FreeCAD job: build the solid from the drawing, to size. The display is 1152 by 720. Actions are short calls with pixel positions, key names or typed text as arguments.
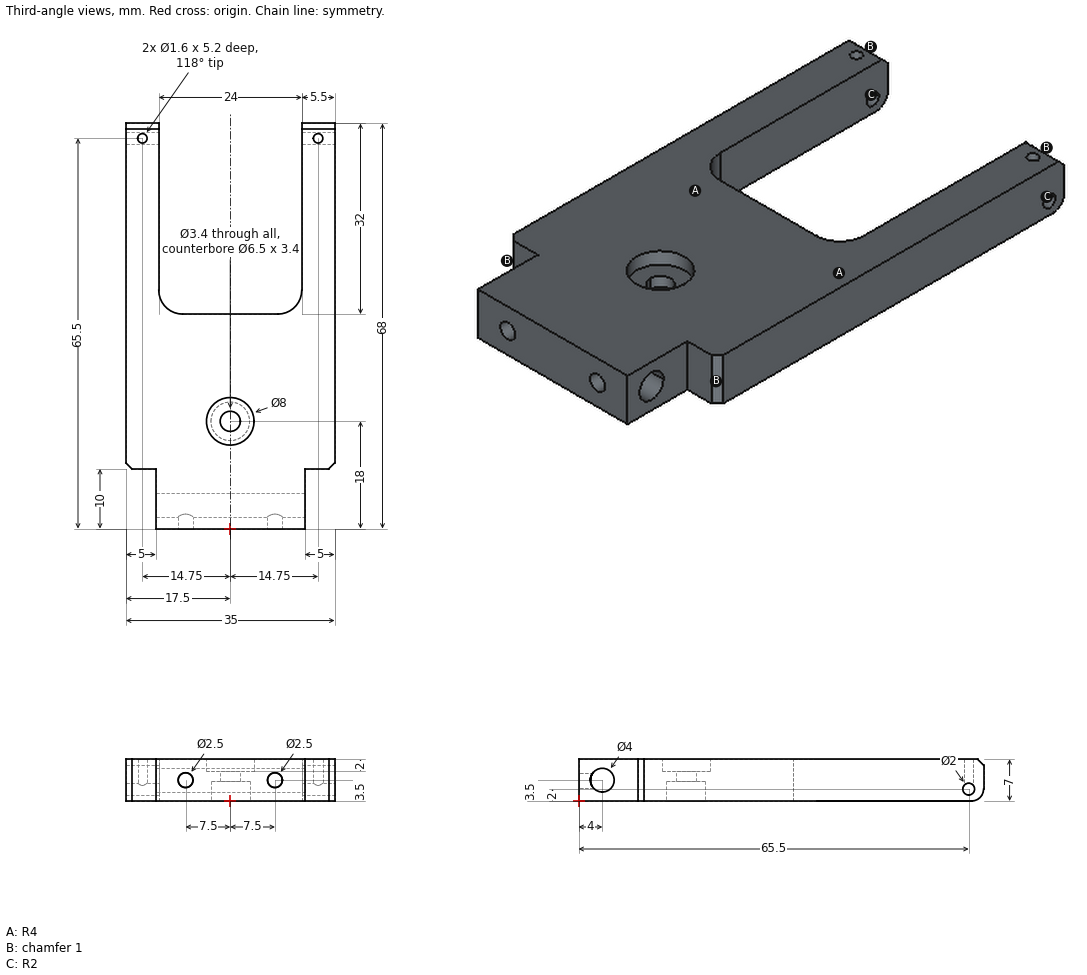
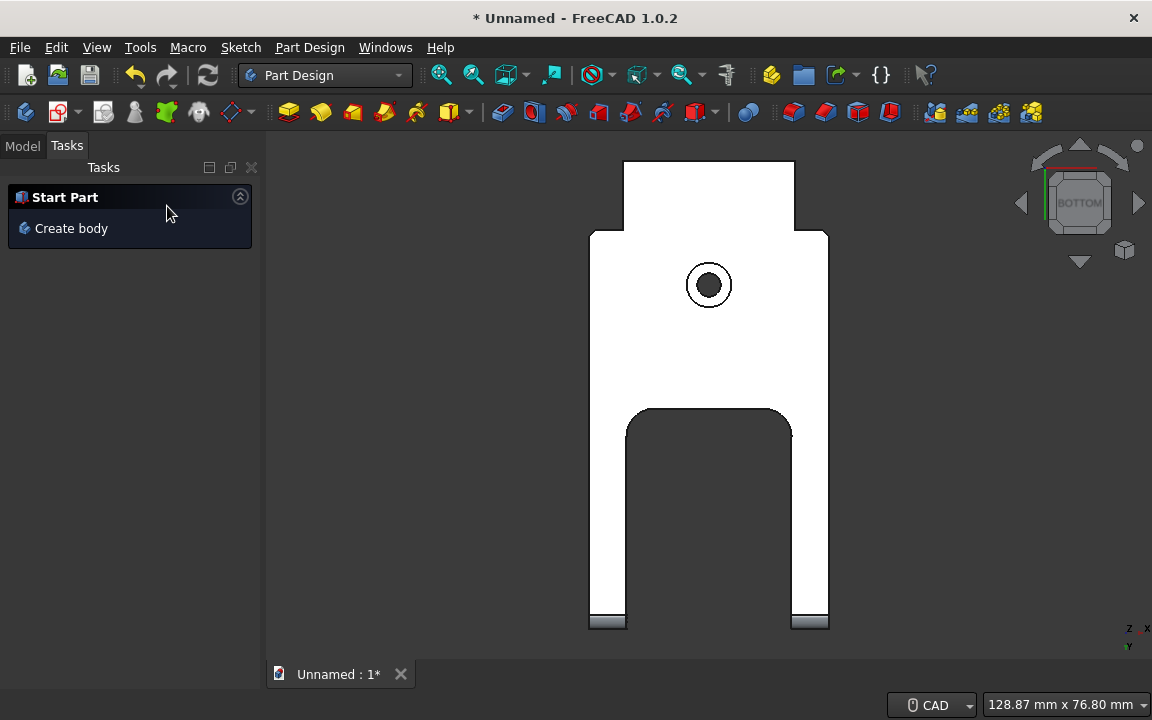
key(0)